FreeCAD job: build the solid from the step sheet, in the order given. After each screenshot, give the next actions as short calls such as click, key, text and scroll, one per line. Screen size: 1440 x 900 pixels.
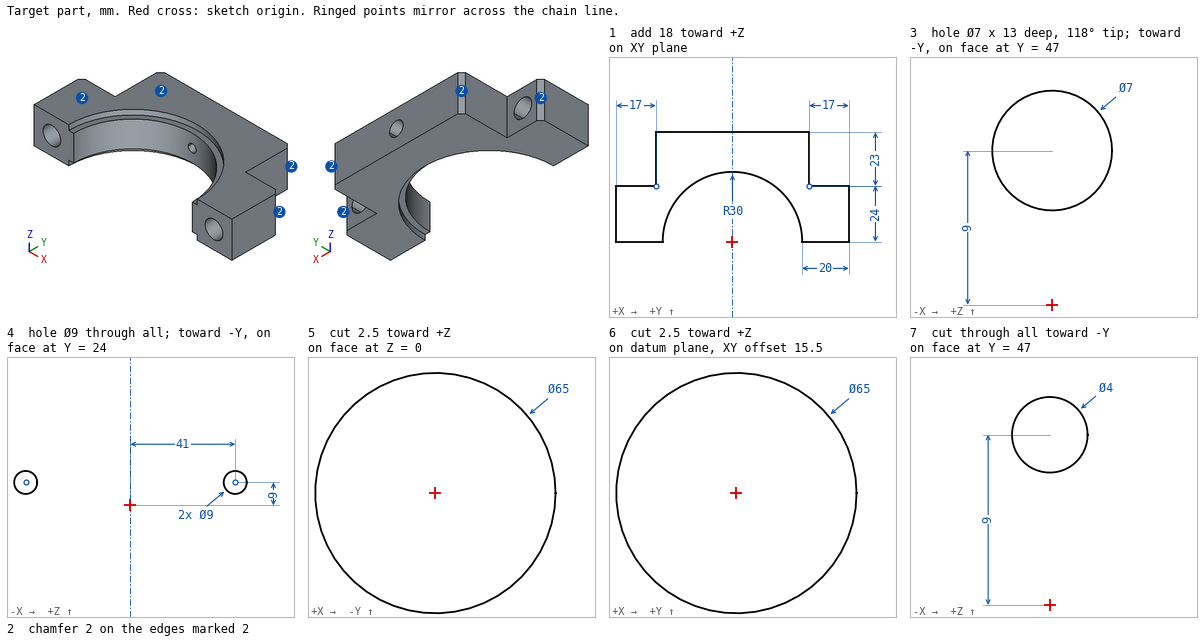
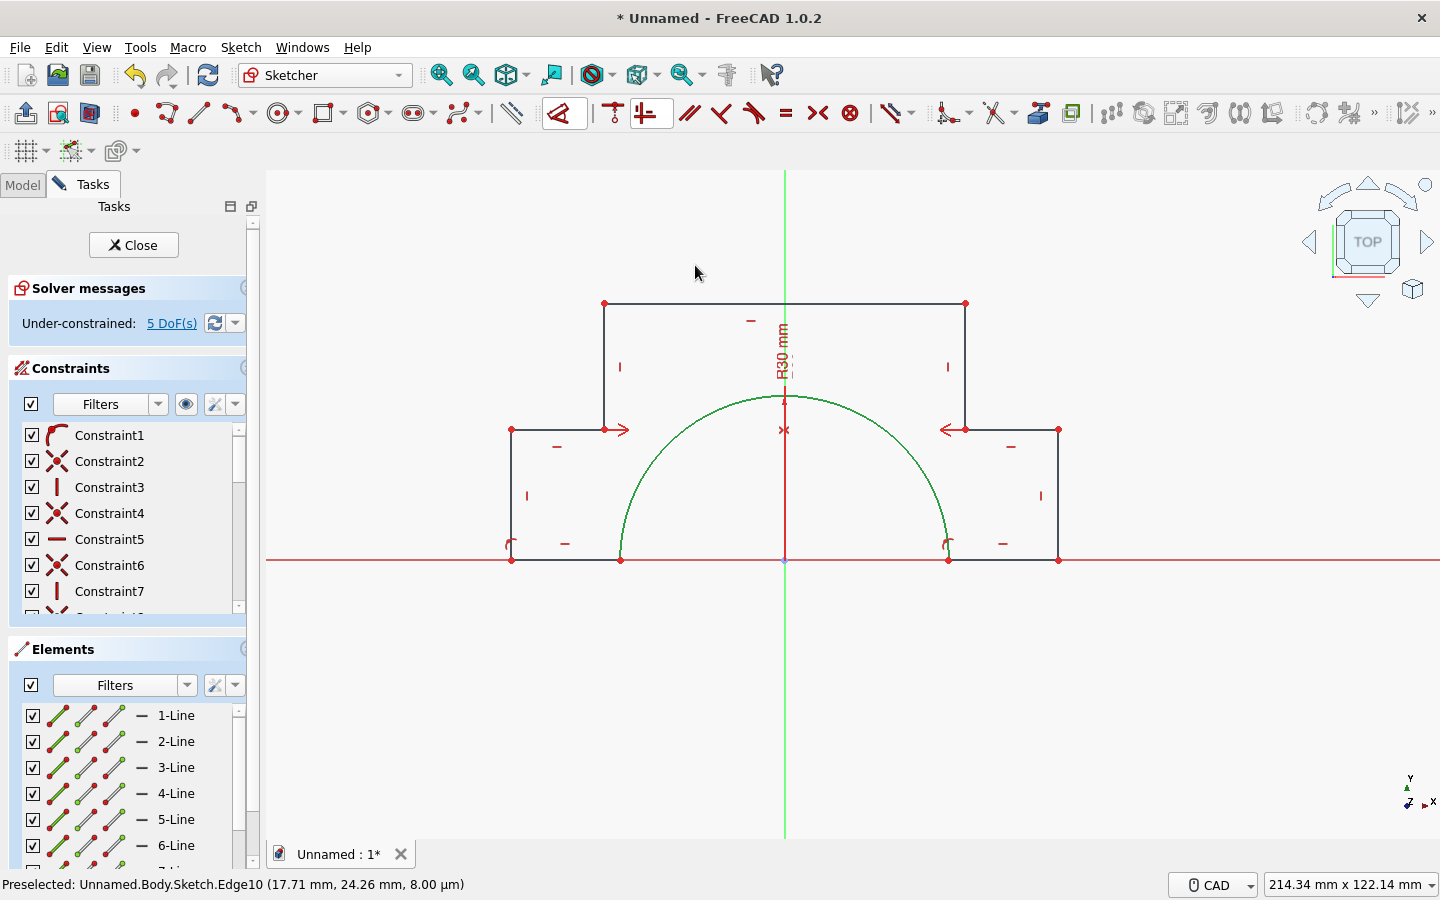
click(982, 560)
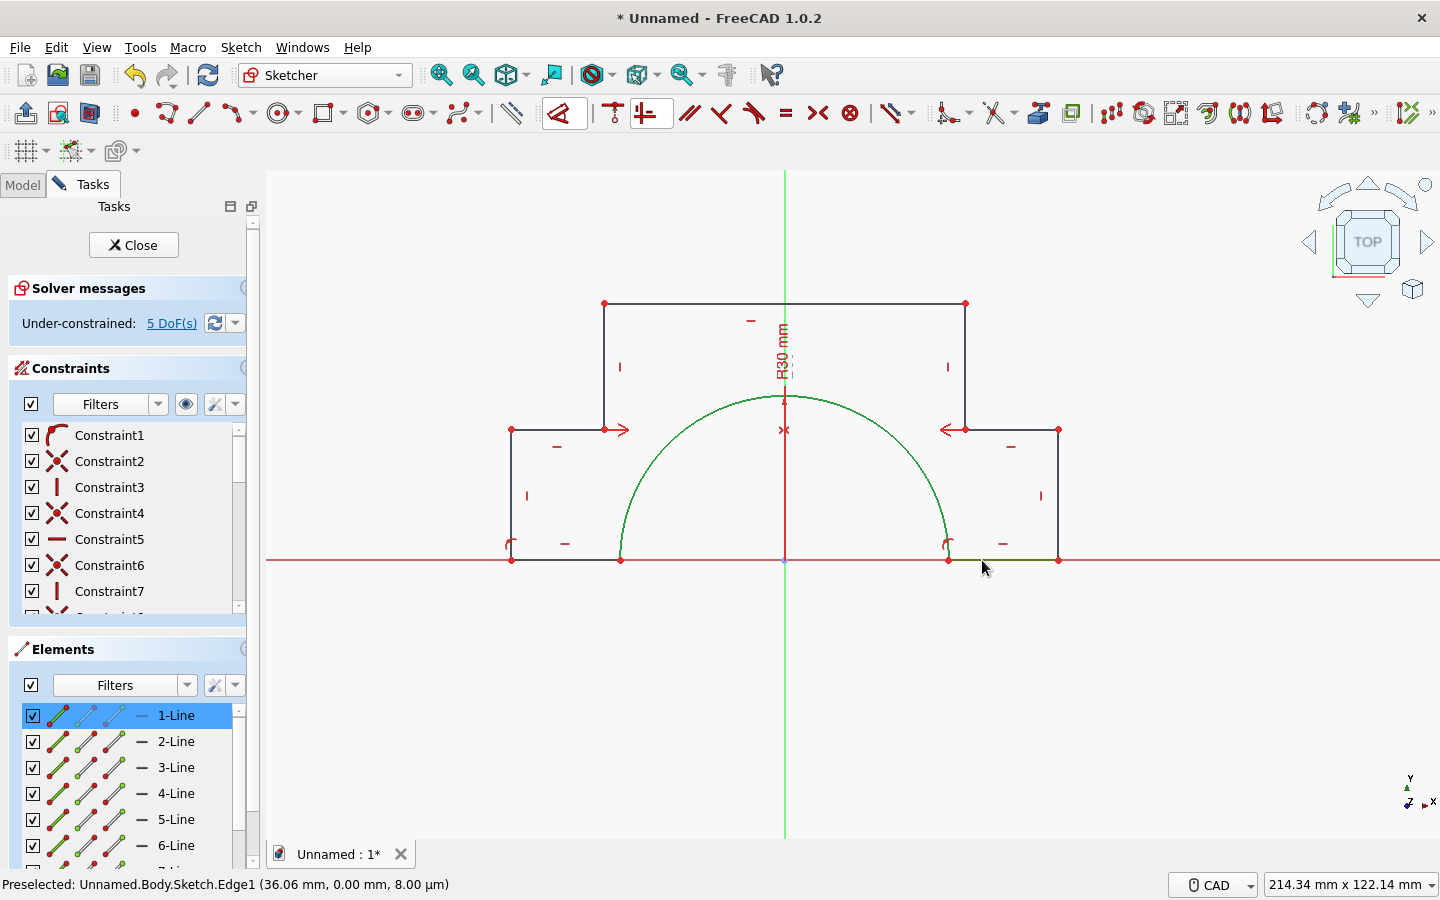
click(582, 114)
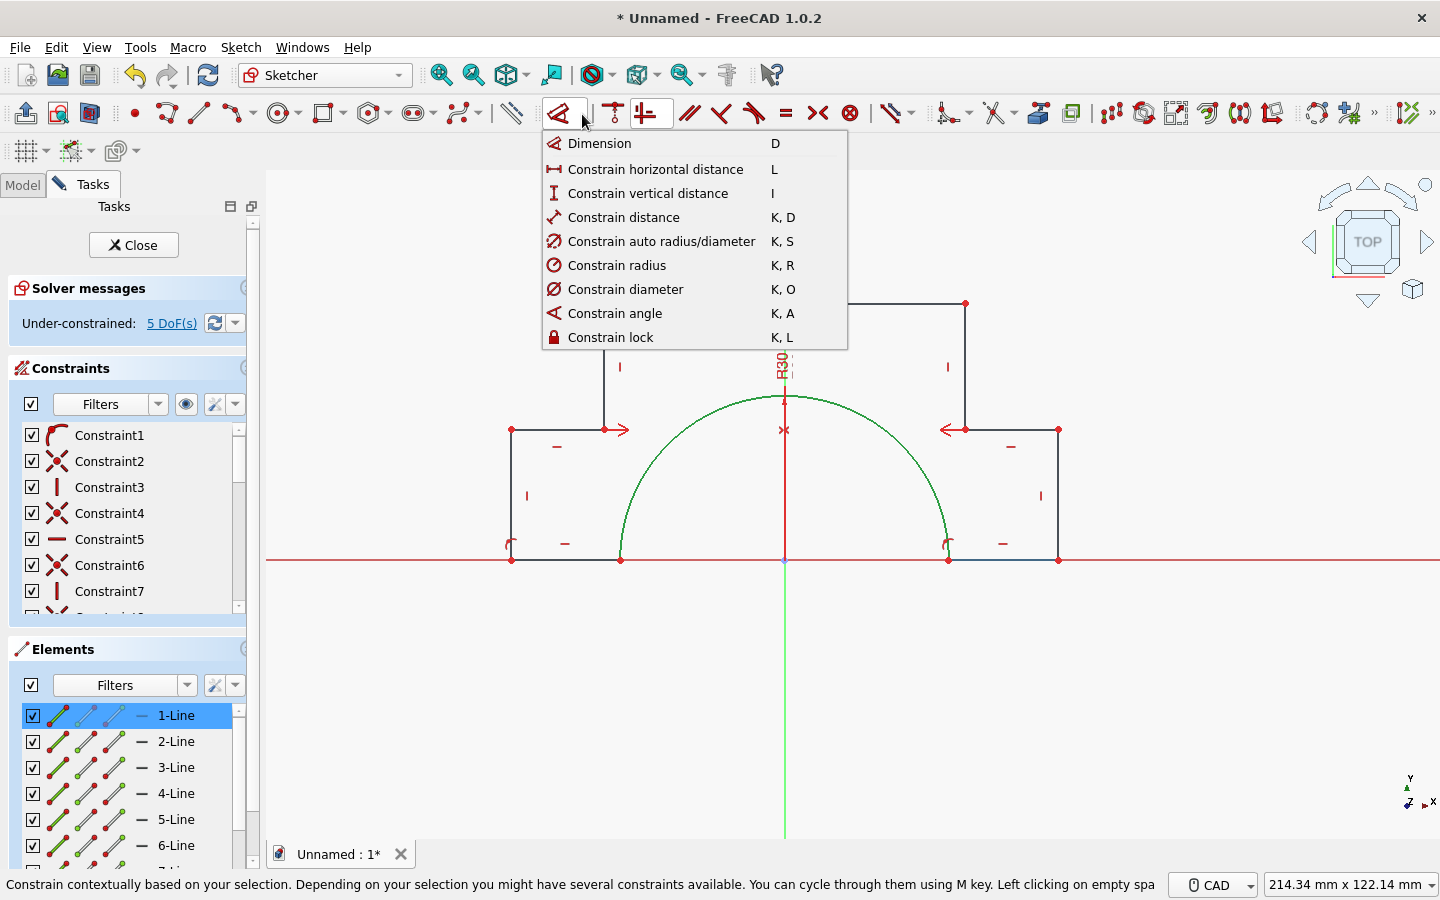
click(695, 169)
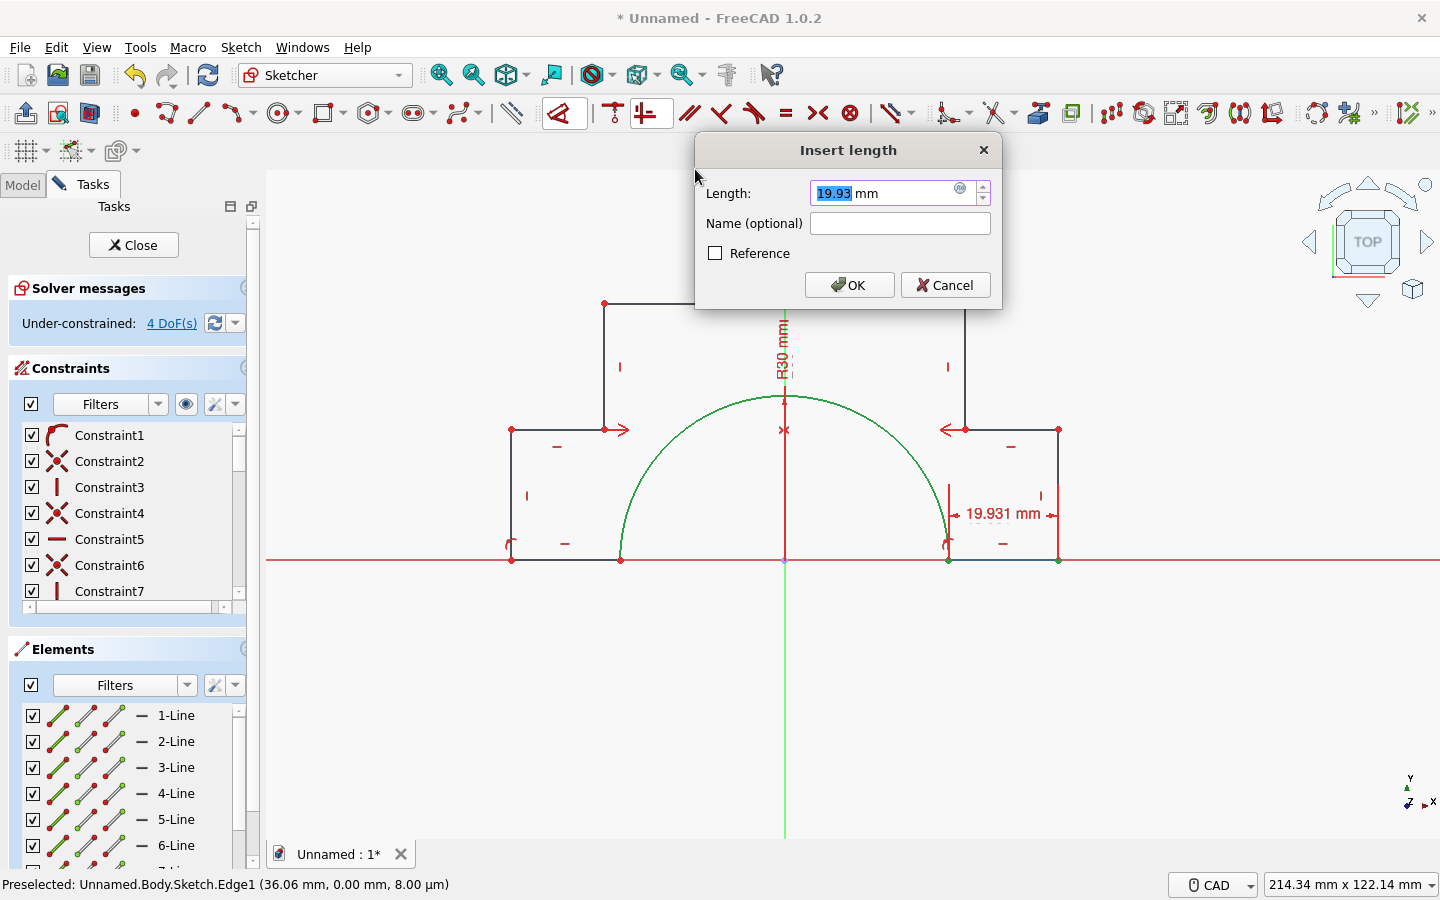
text(20)
key(Return)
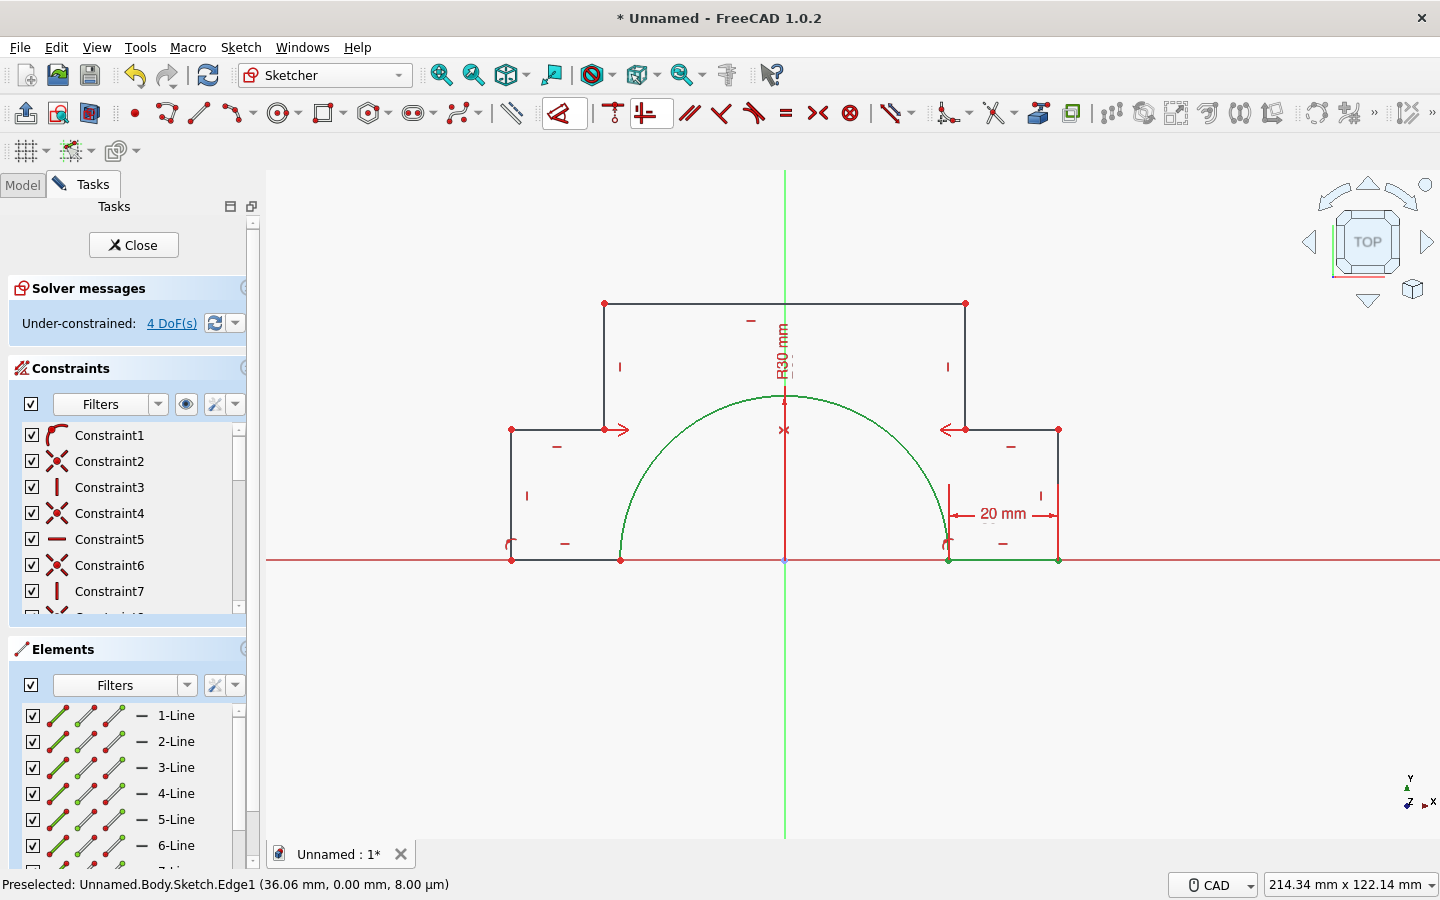
click(1058, 521)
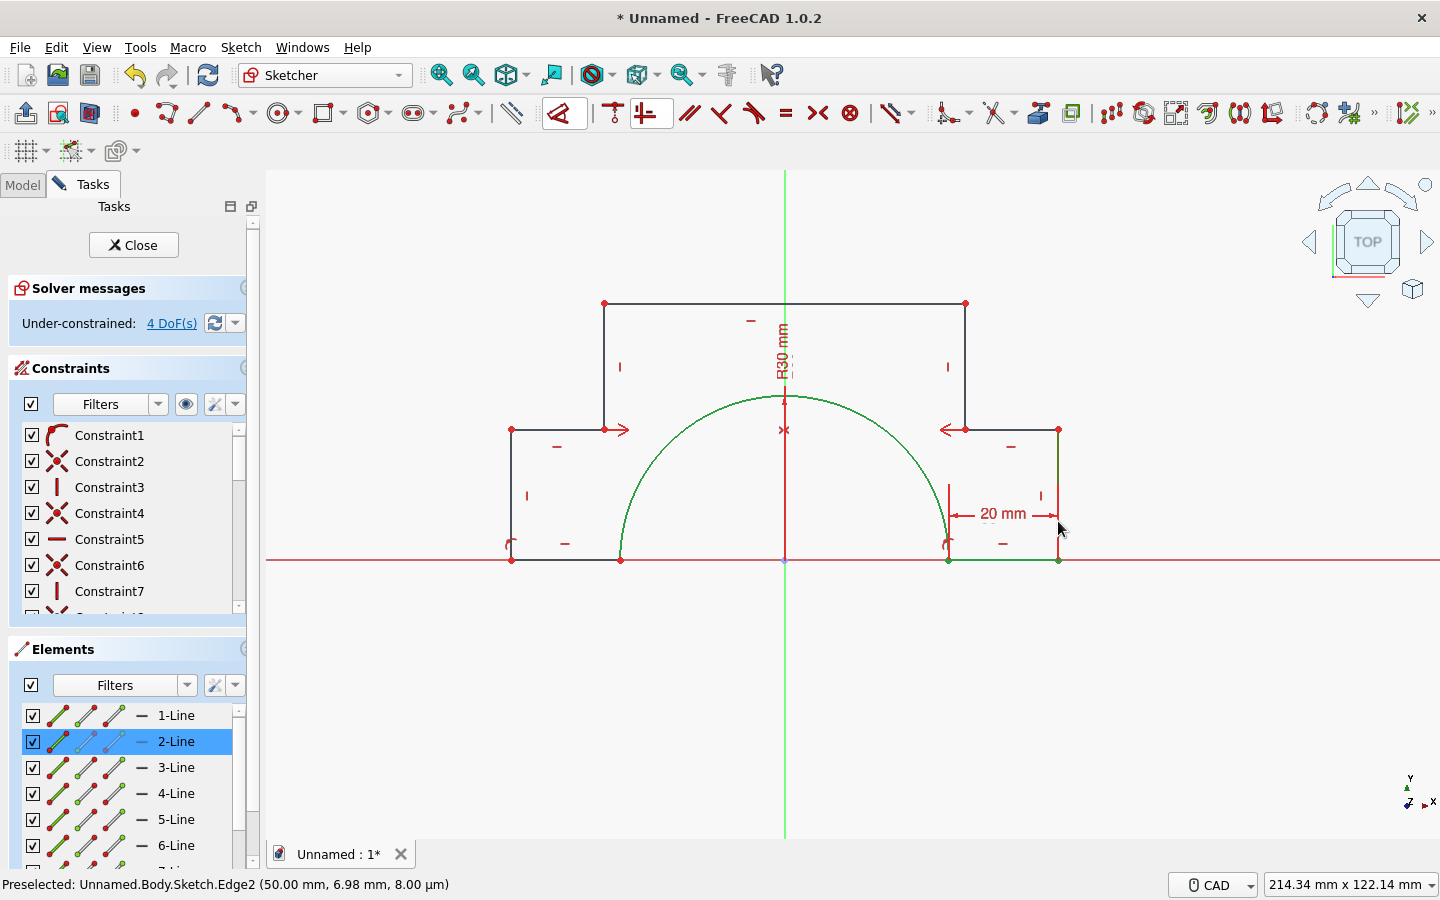
key(i)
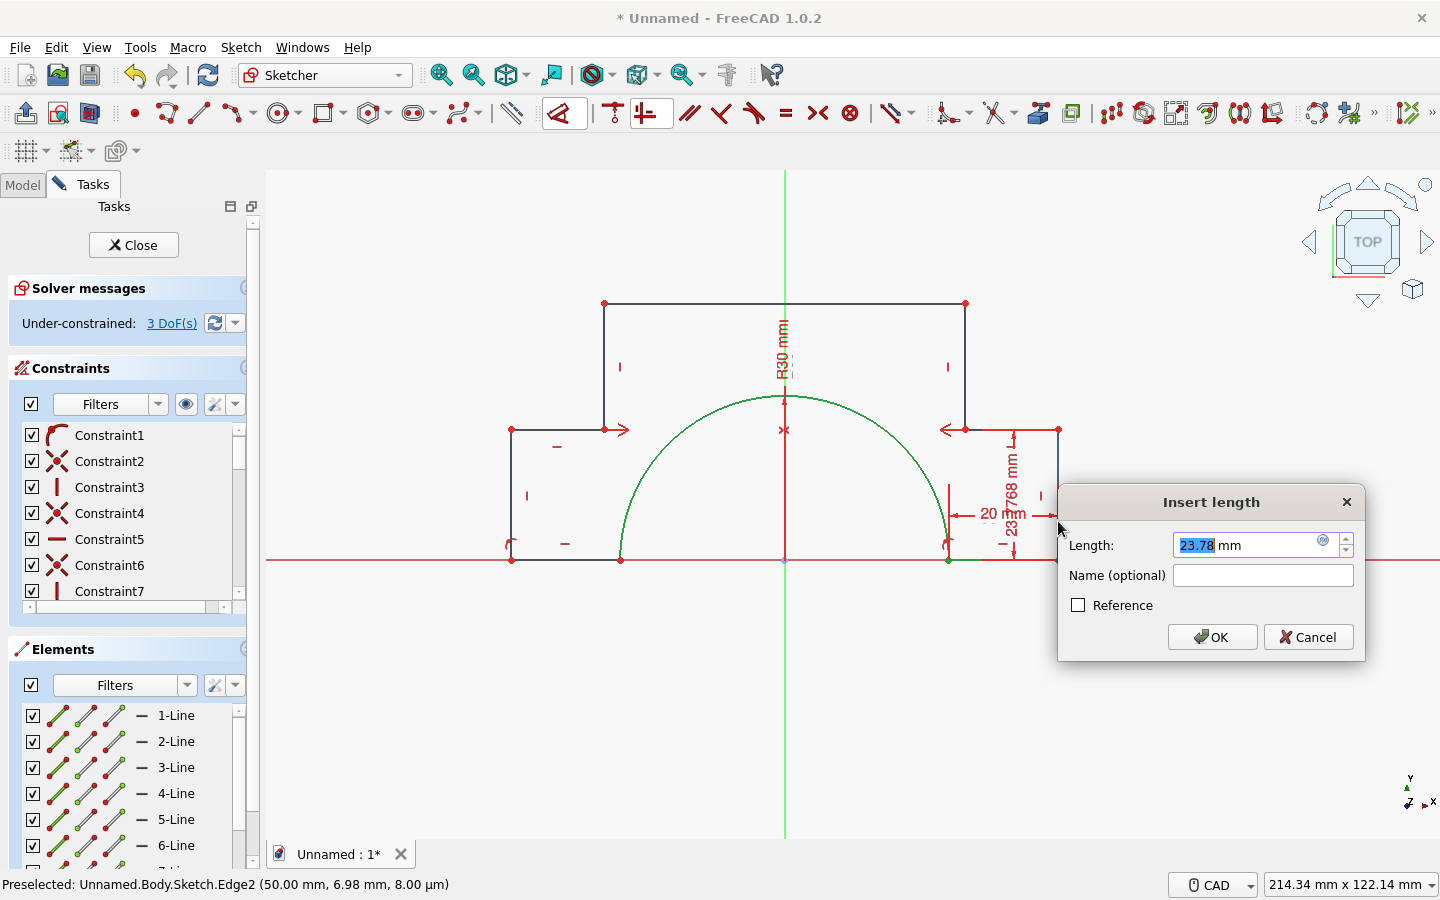
text(24)
key(Return)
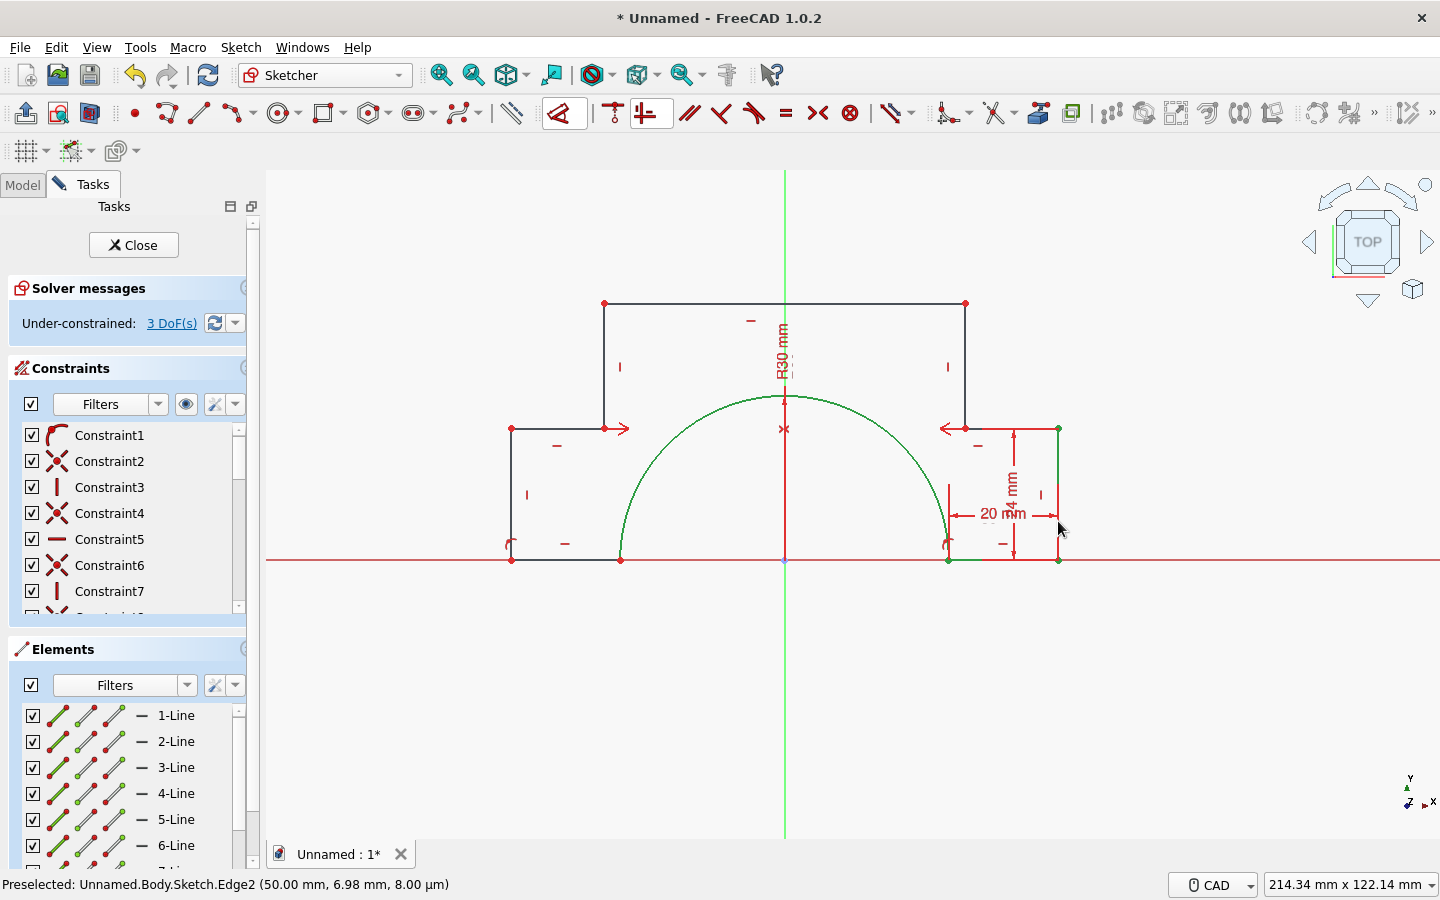
click(1030, 429)